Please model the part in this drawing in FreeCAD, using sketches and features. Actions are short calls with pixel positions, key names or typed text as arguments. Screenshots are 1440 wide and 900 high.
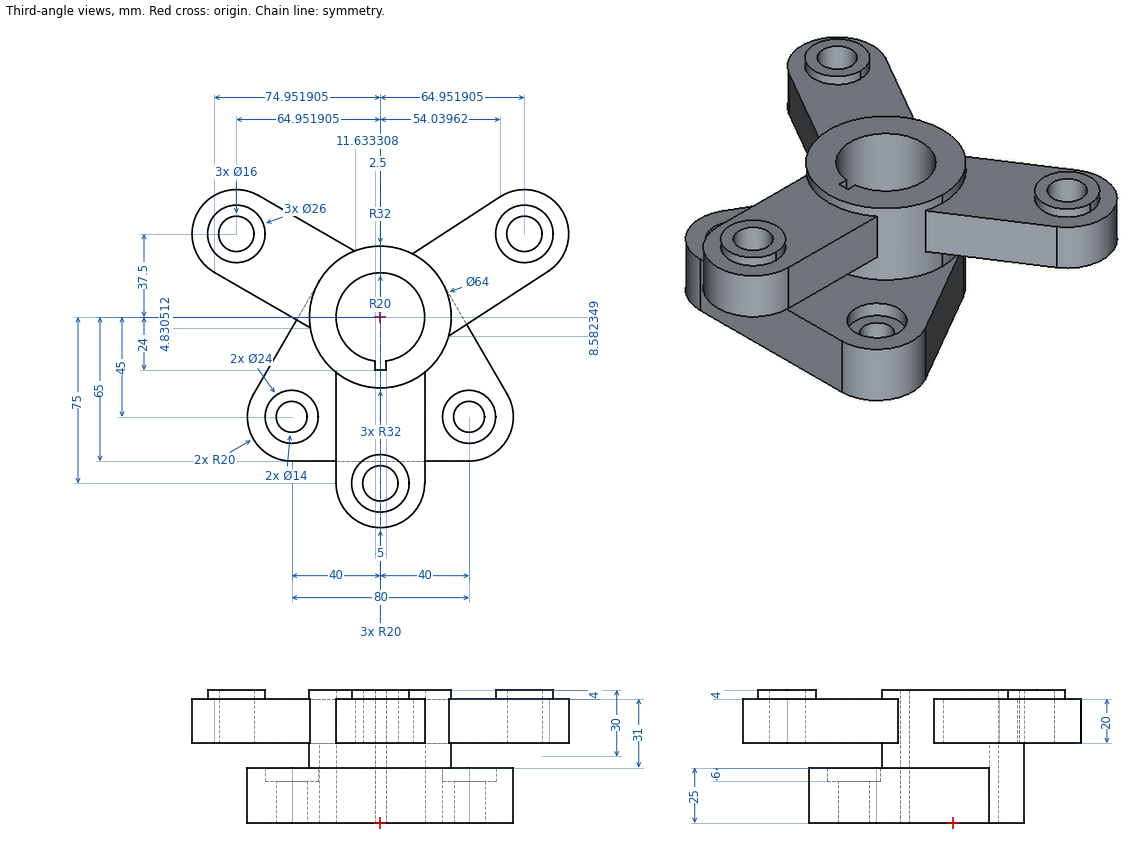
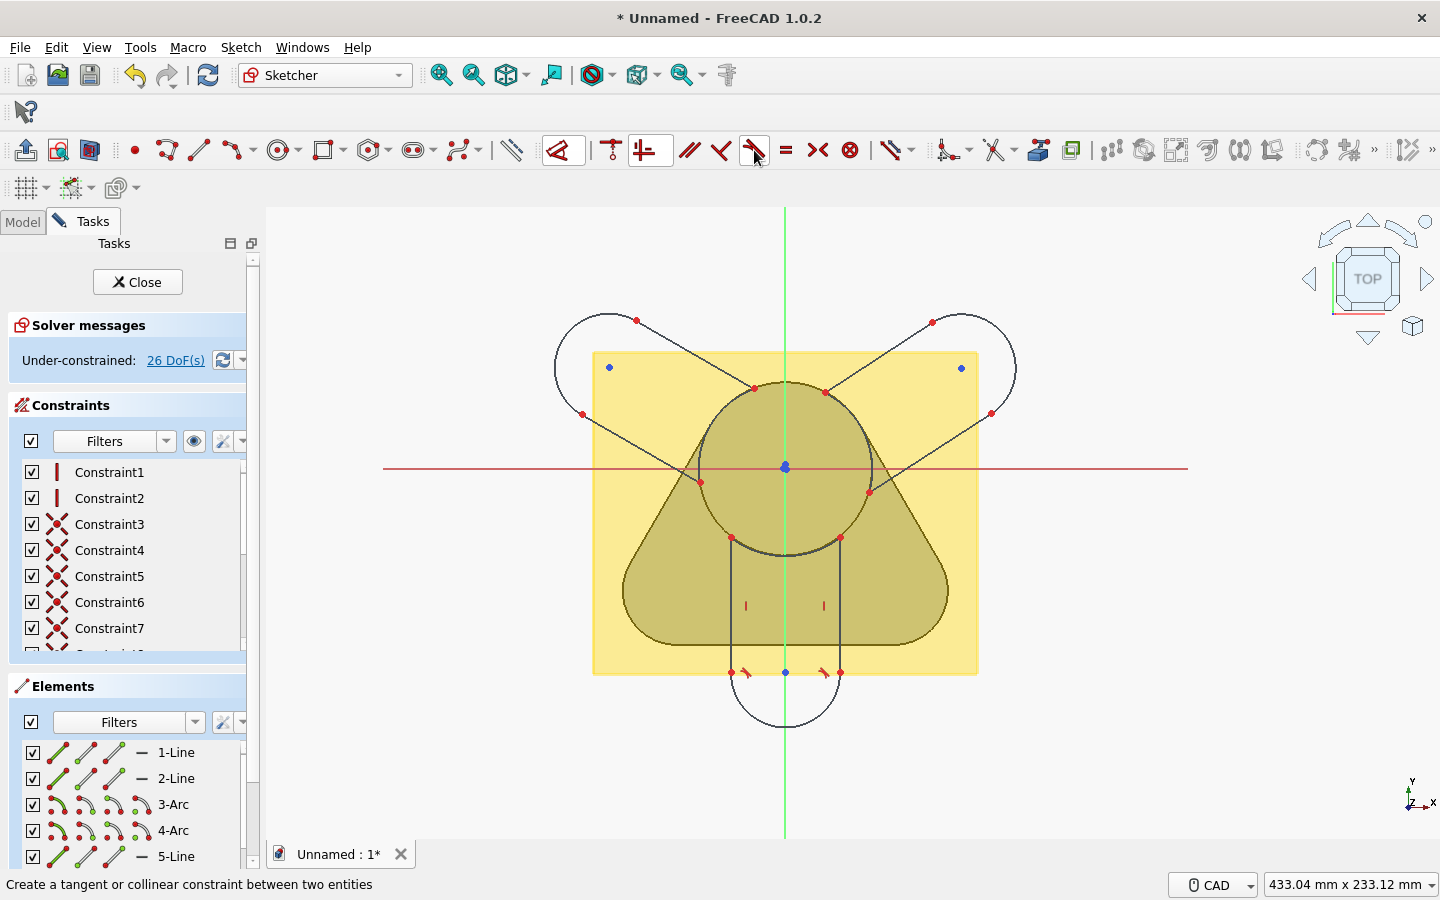
click(617, 435)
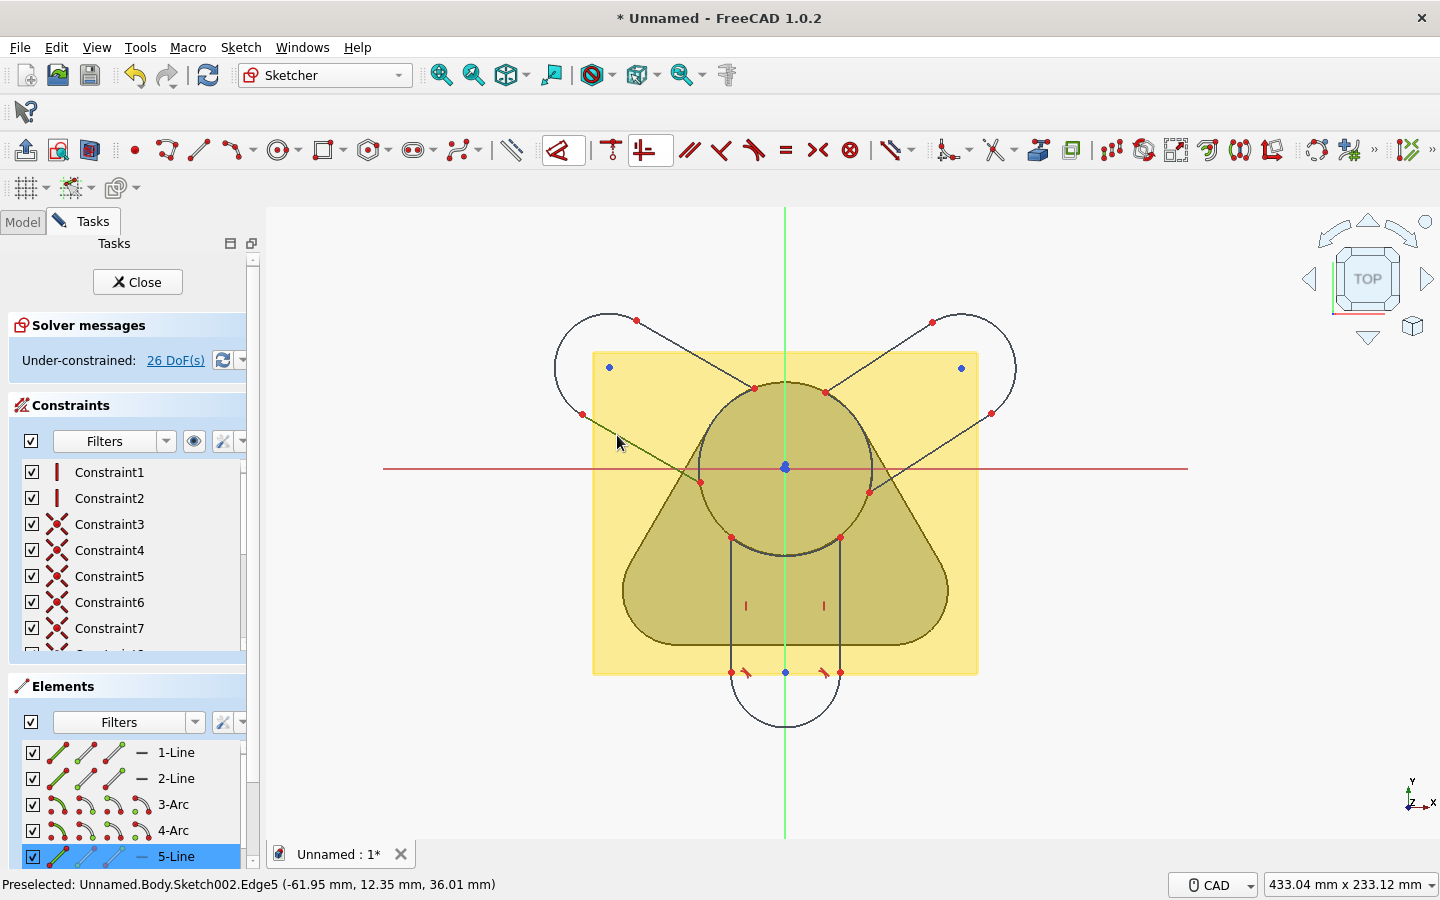
click(587, 319)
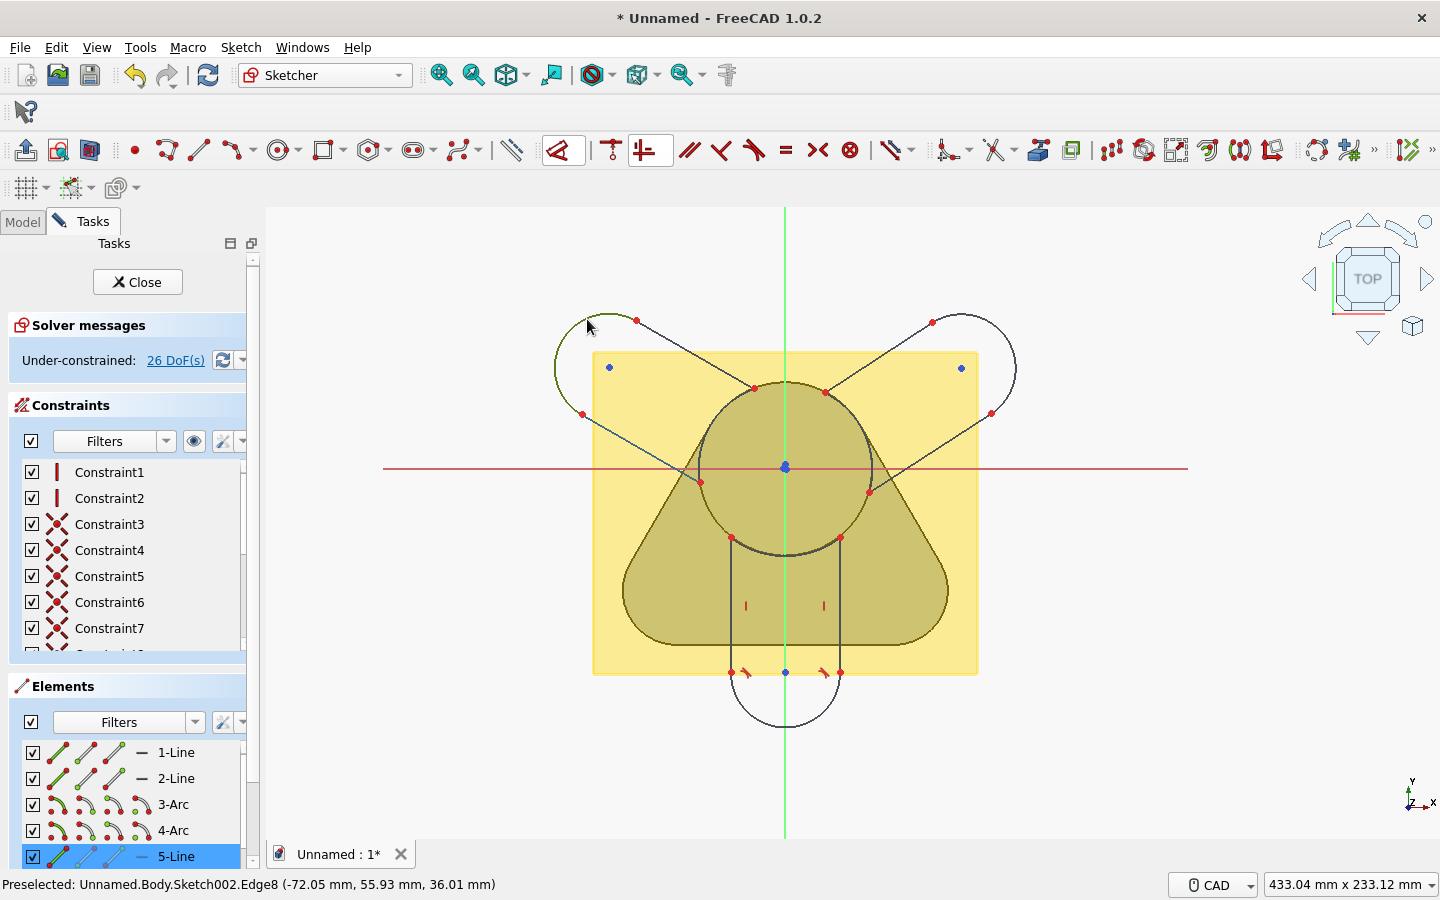
click(754, 150)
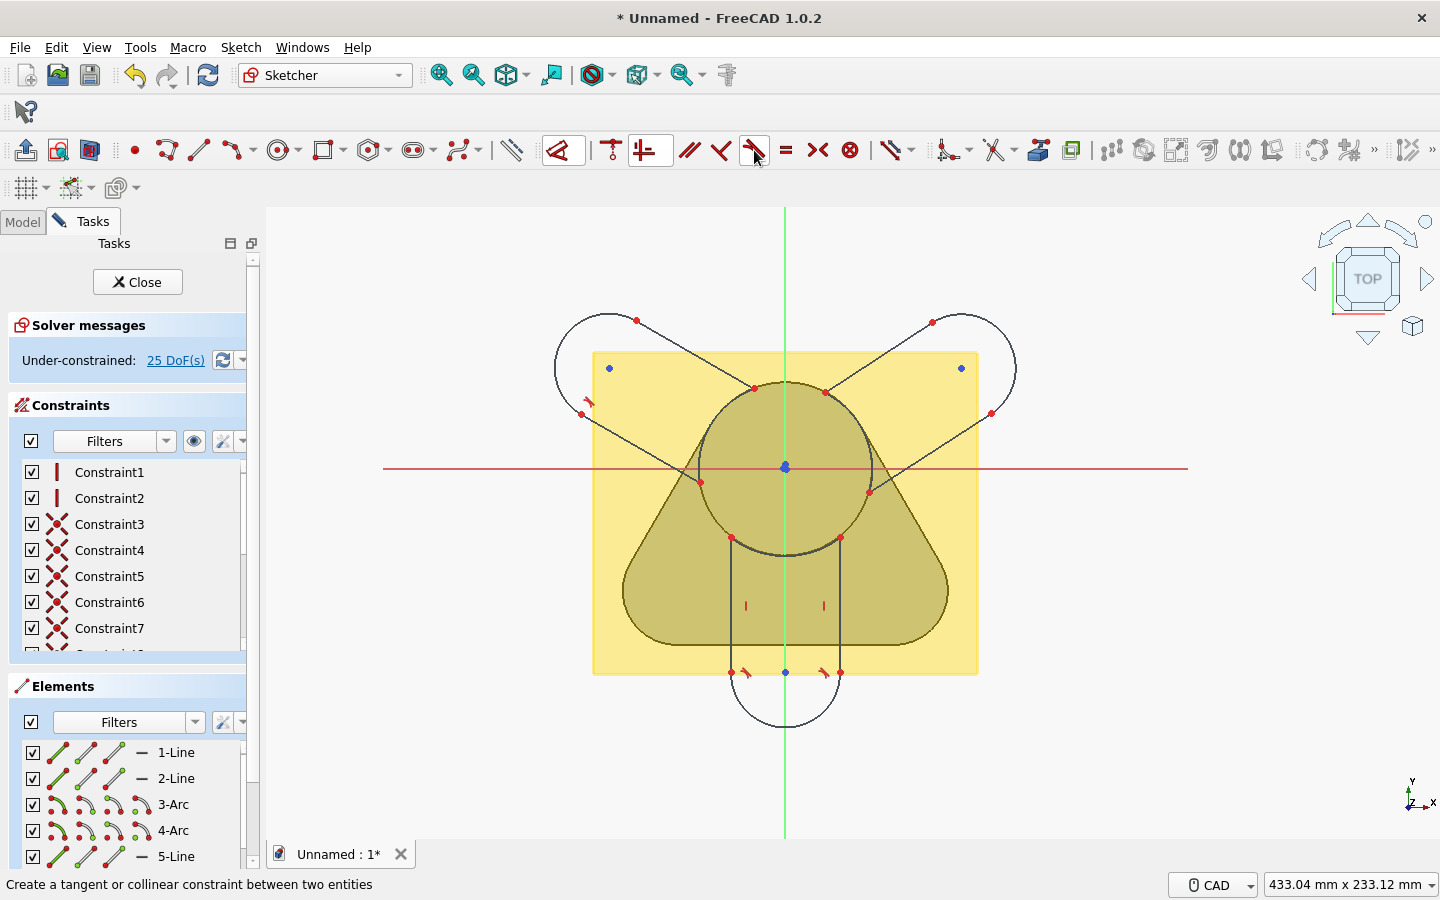
click(719, 369)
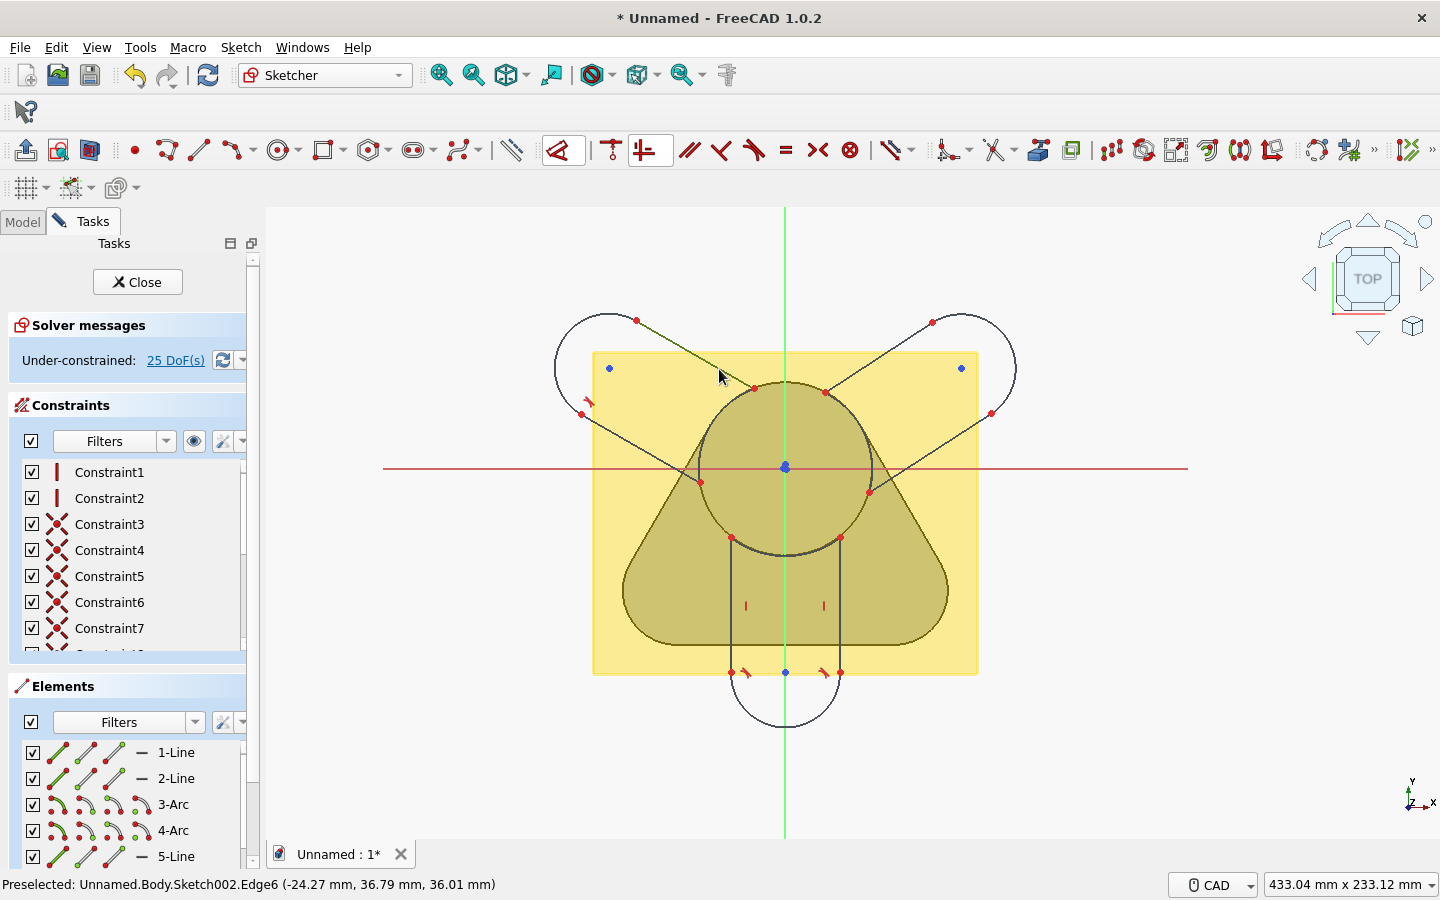
click(587, 319)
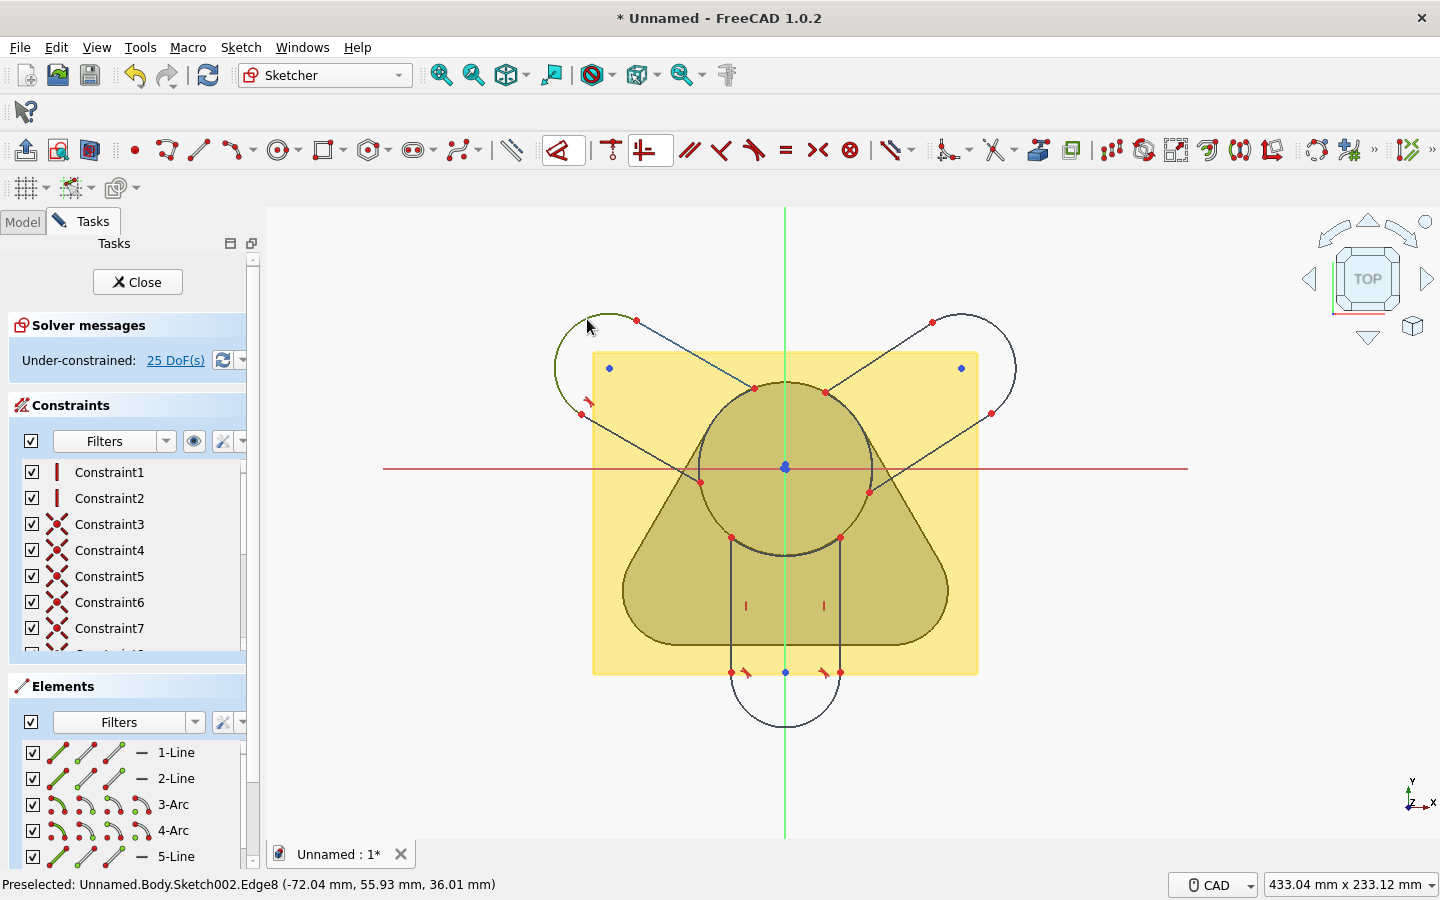
click(754, 150)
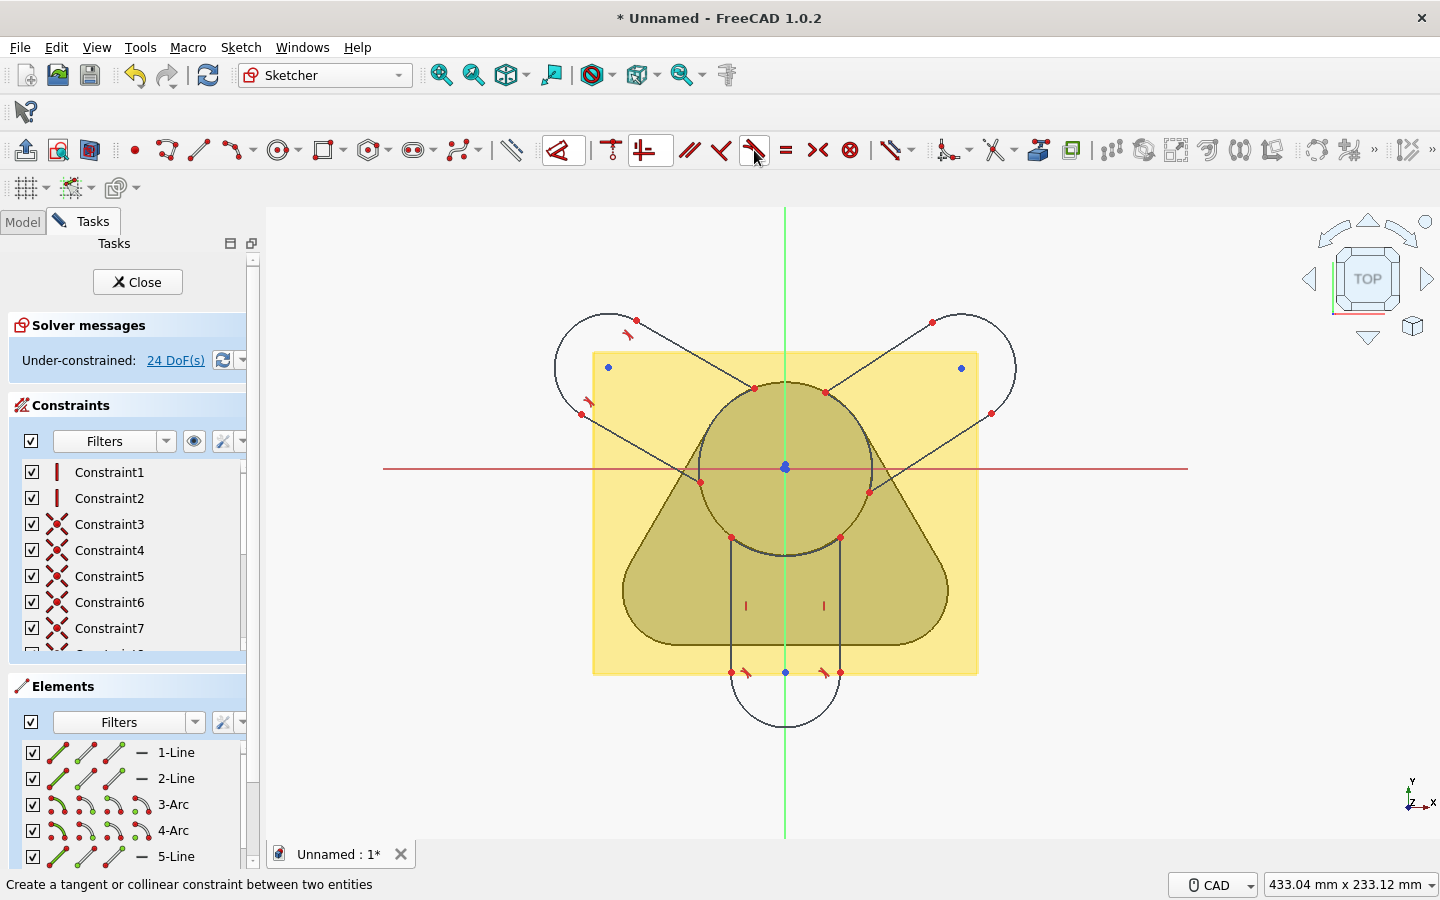
click(900, 344)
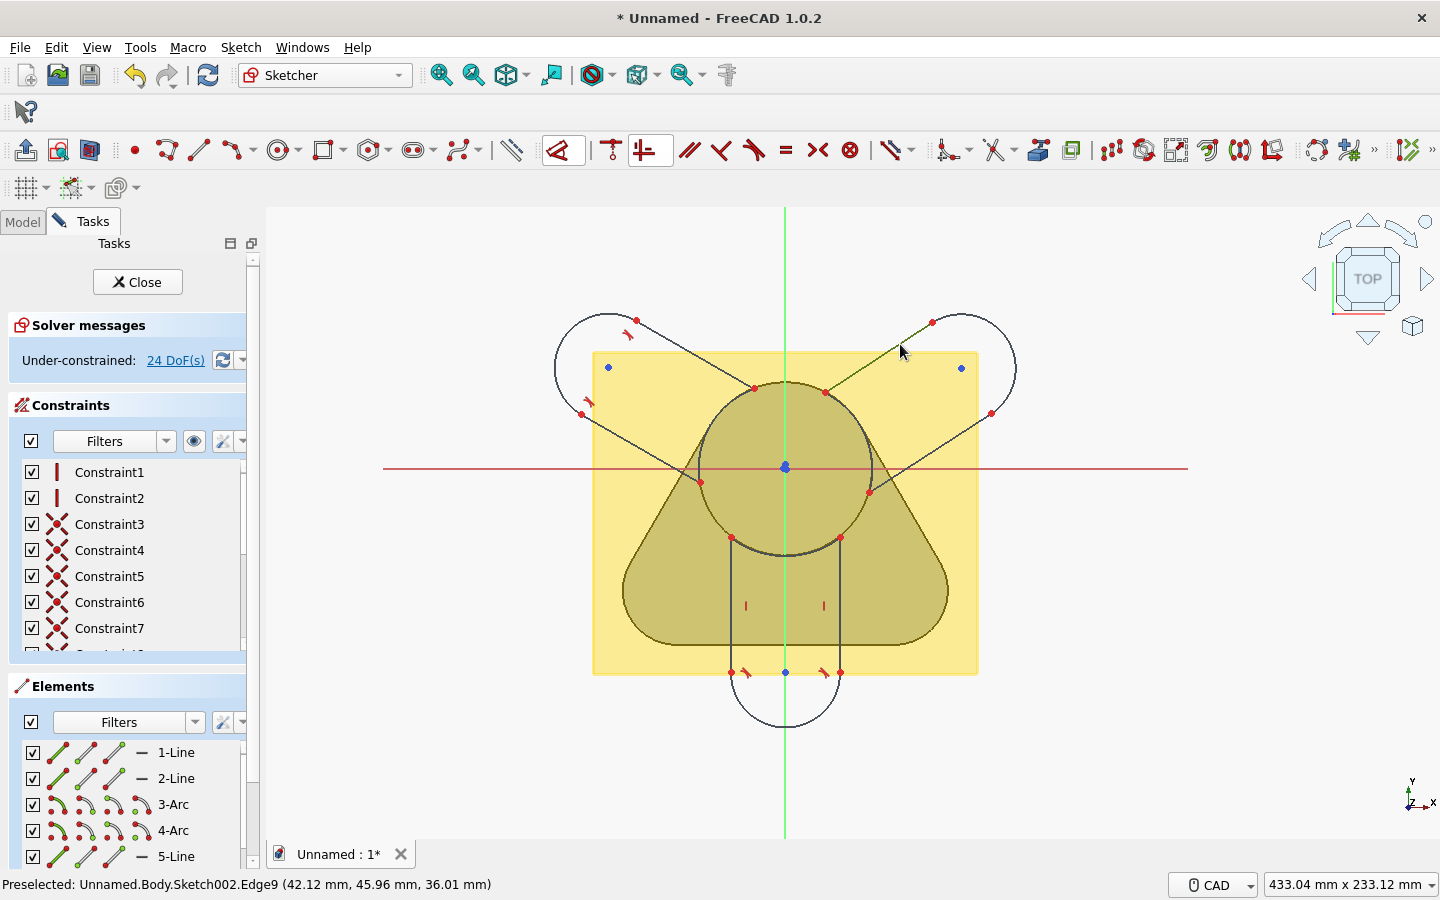
click(1016, 371)